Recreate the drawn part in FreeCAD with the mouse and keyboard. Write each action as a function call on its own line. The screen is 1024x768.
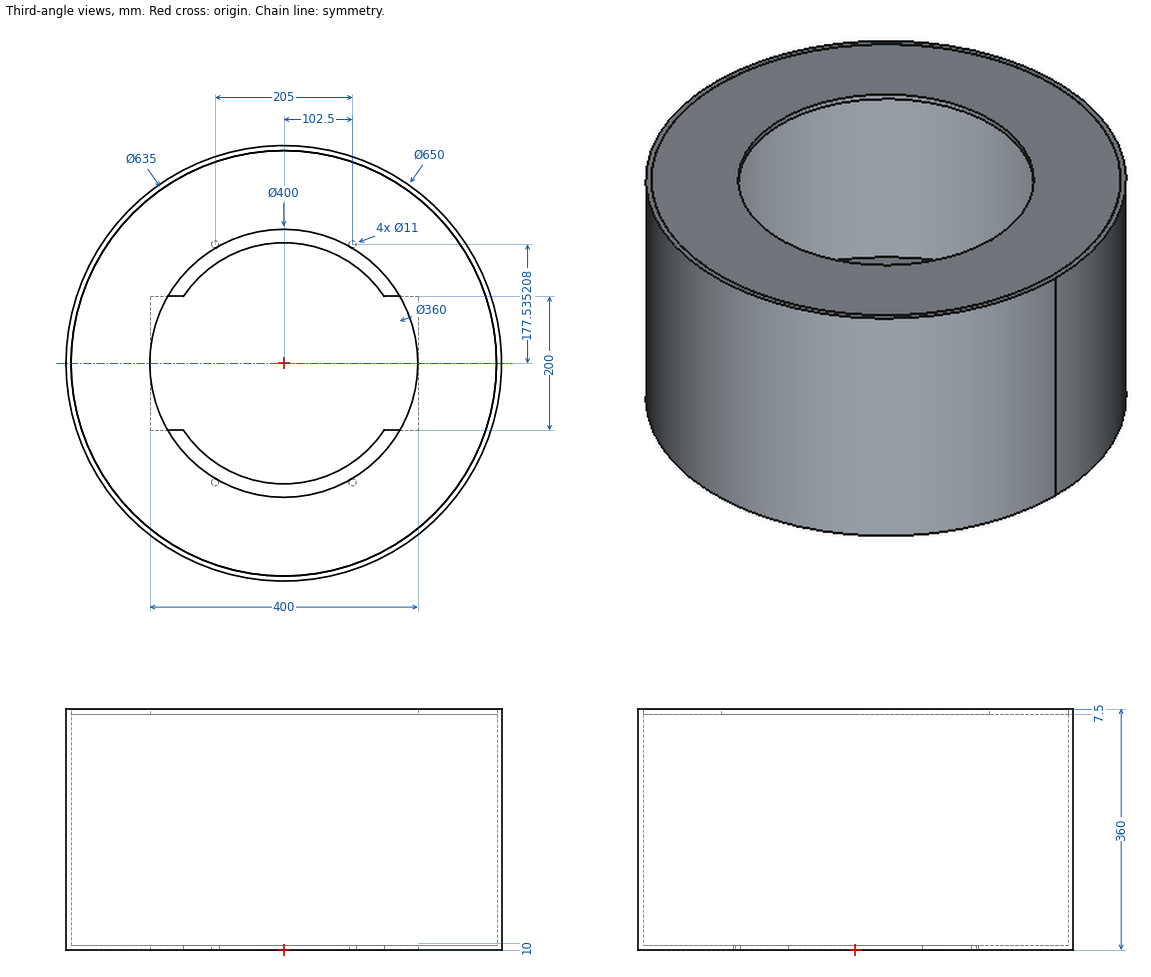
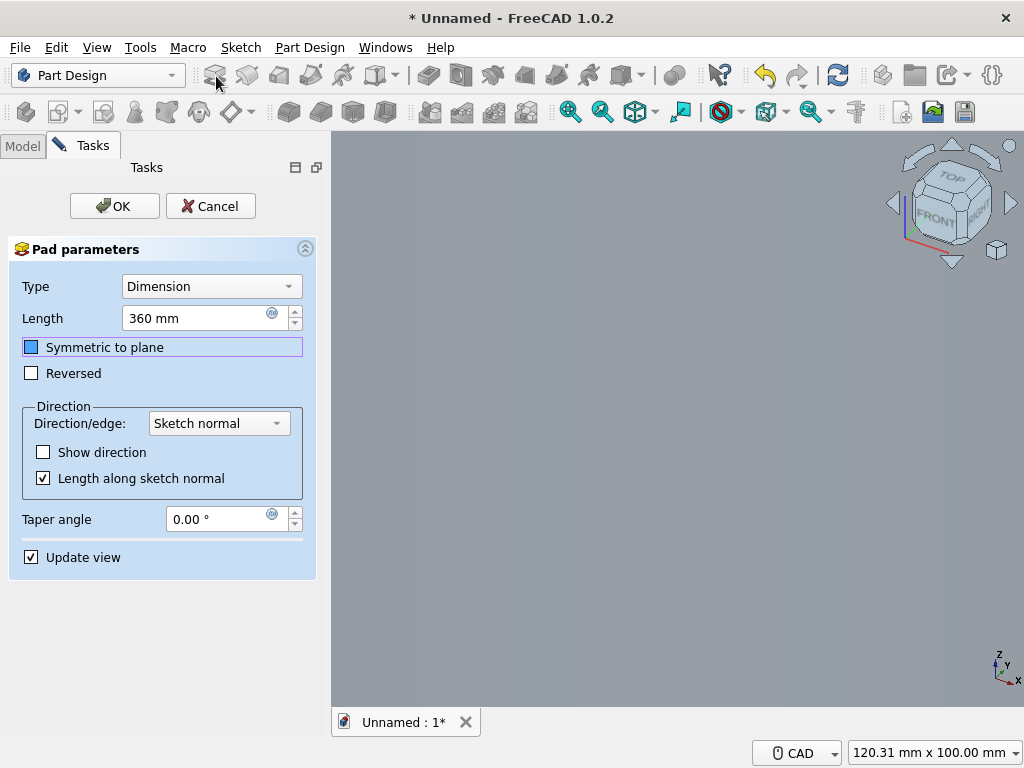
click(115, 206)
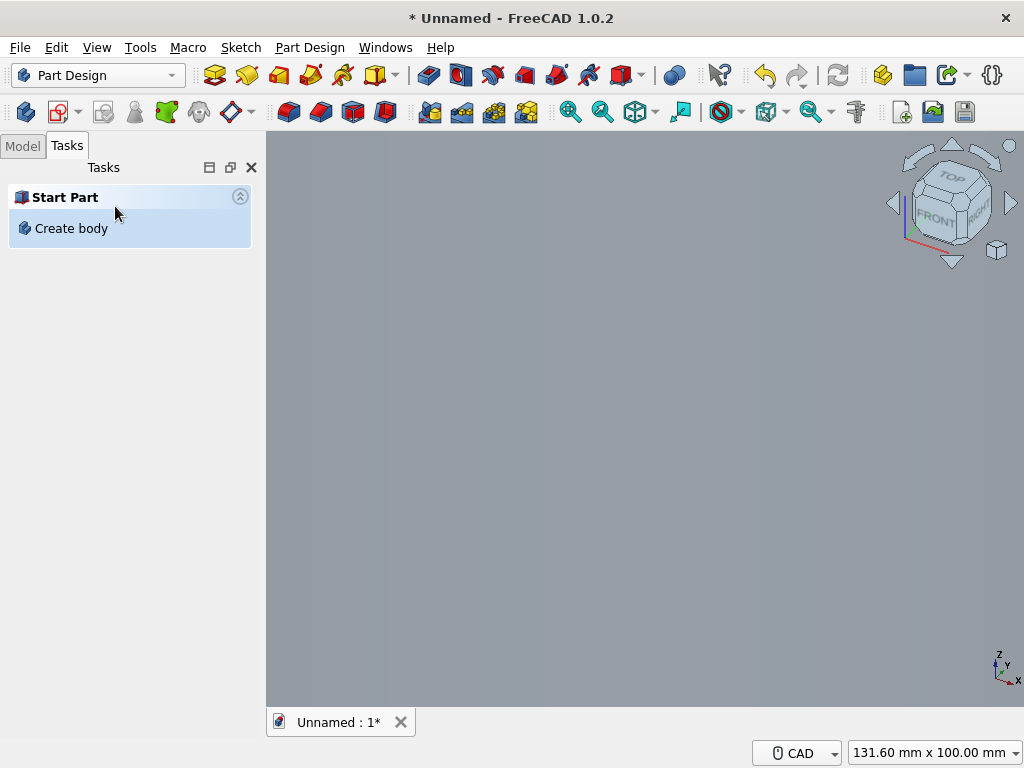
click(572, 112)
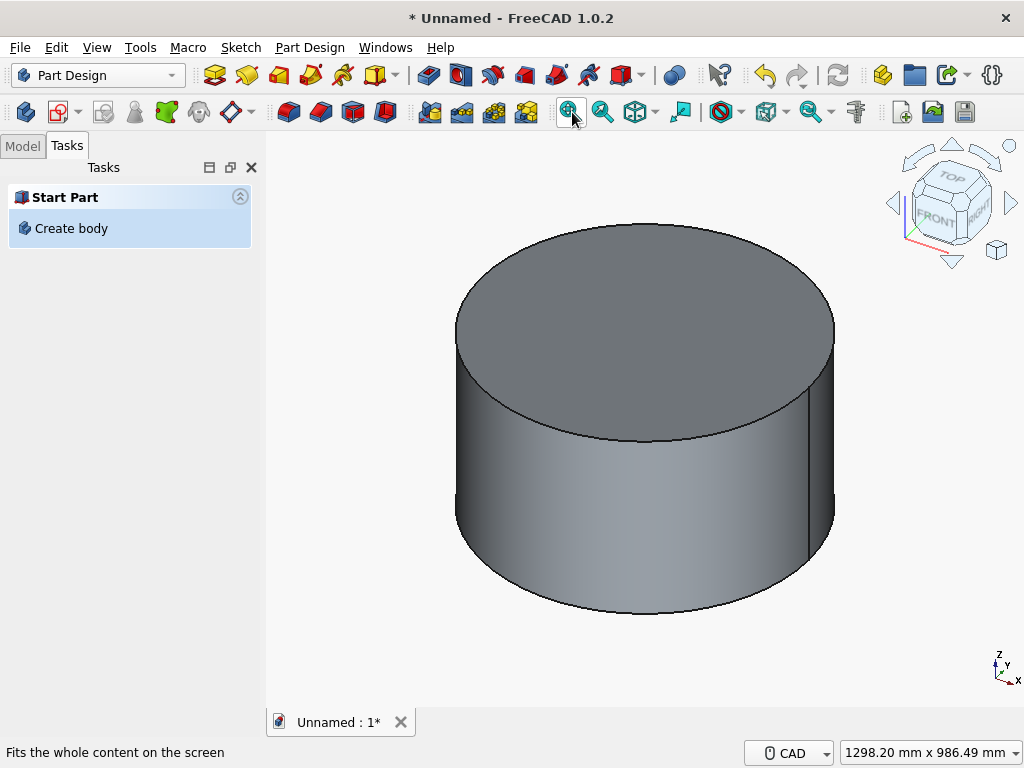
click(58, 112)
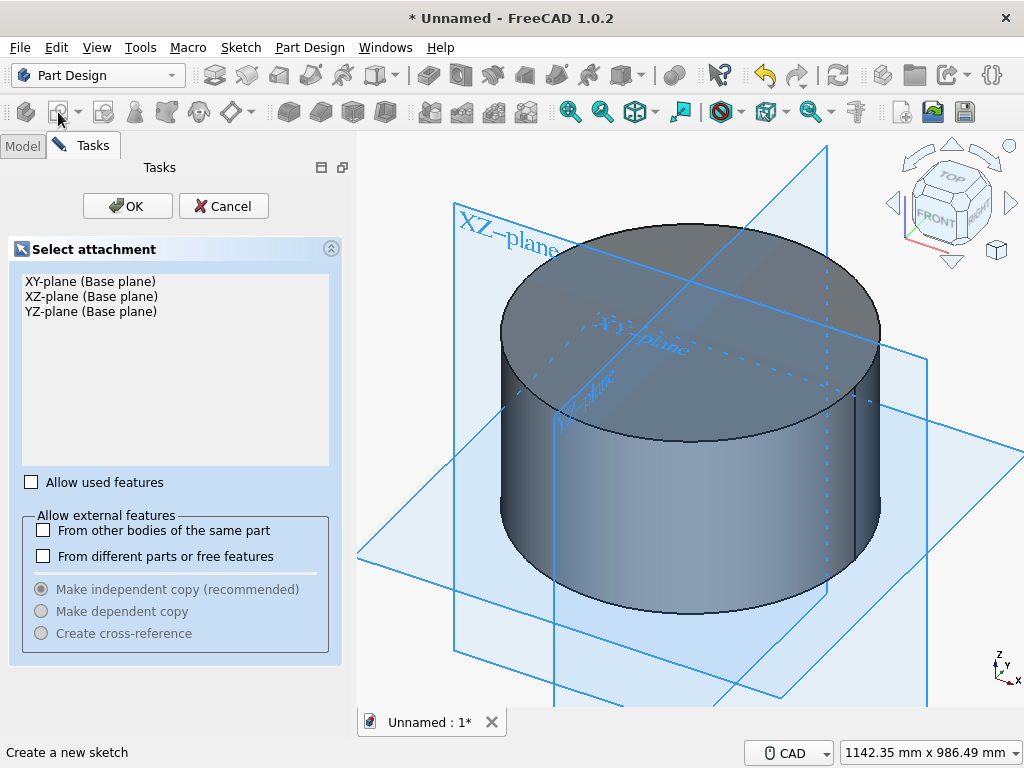
click(82, 282)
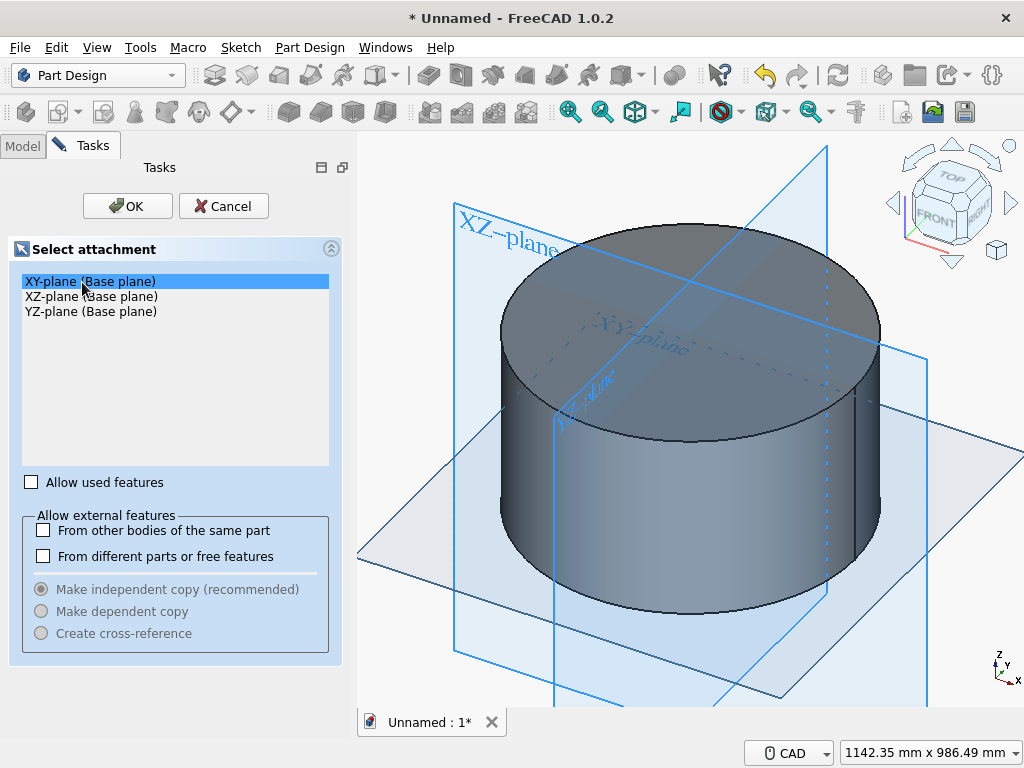
click(128, 206)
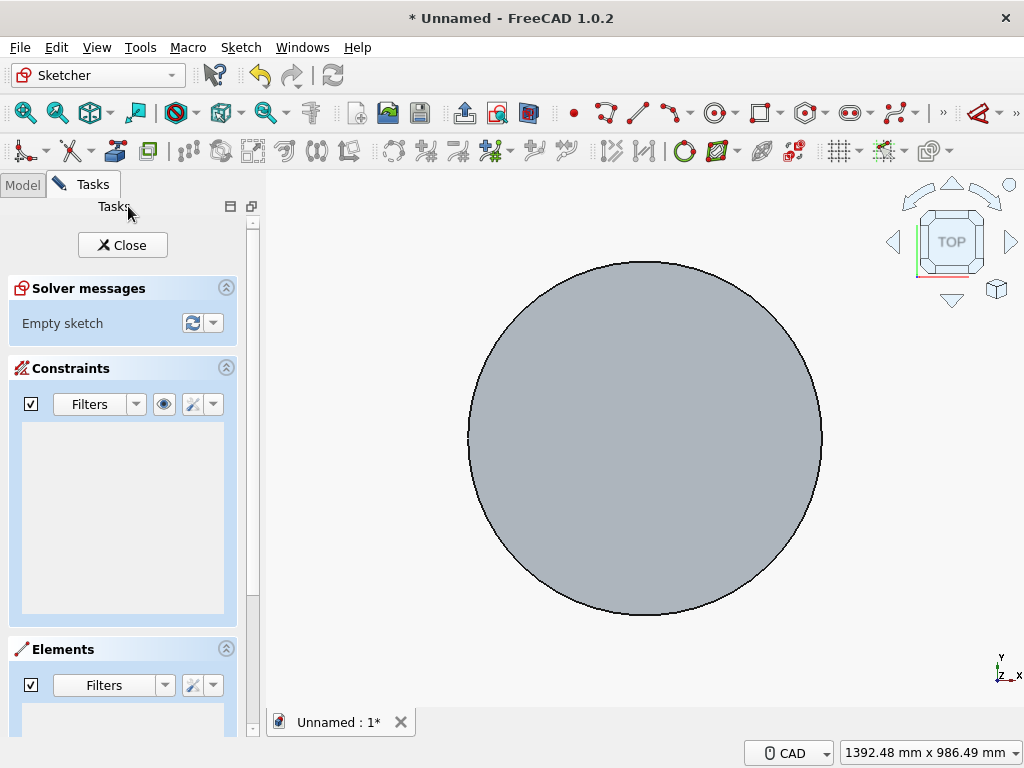
click(530, 114)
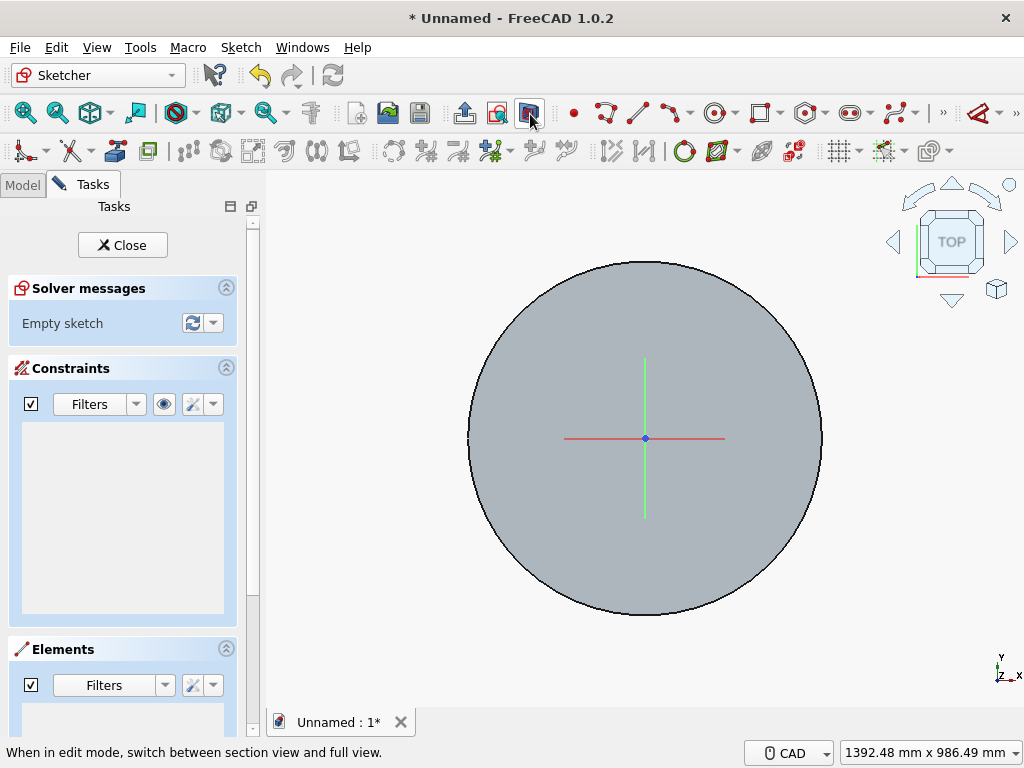
scroll(728, 438, up, 3)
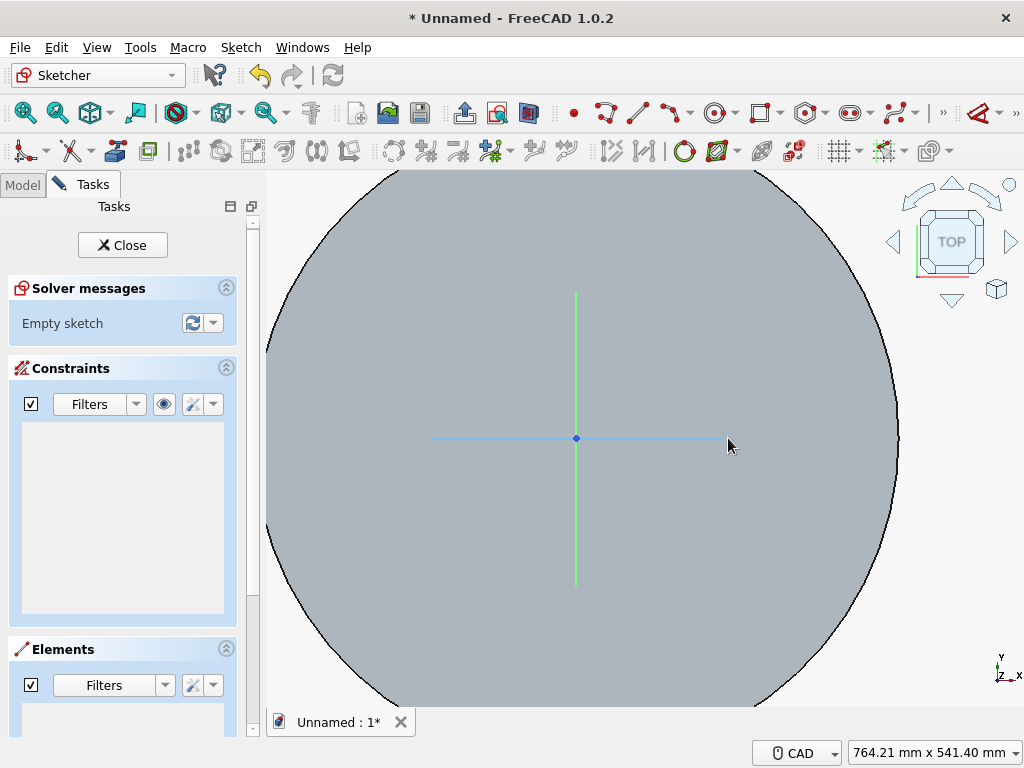
click(716, 114)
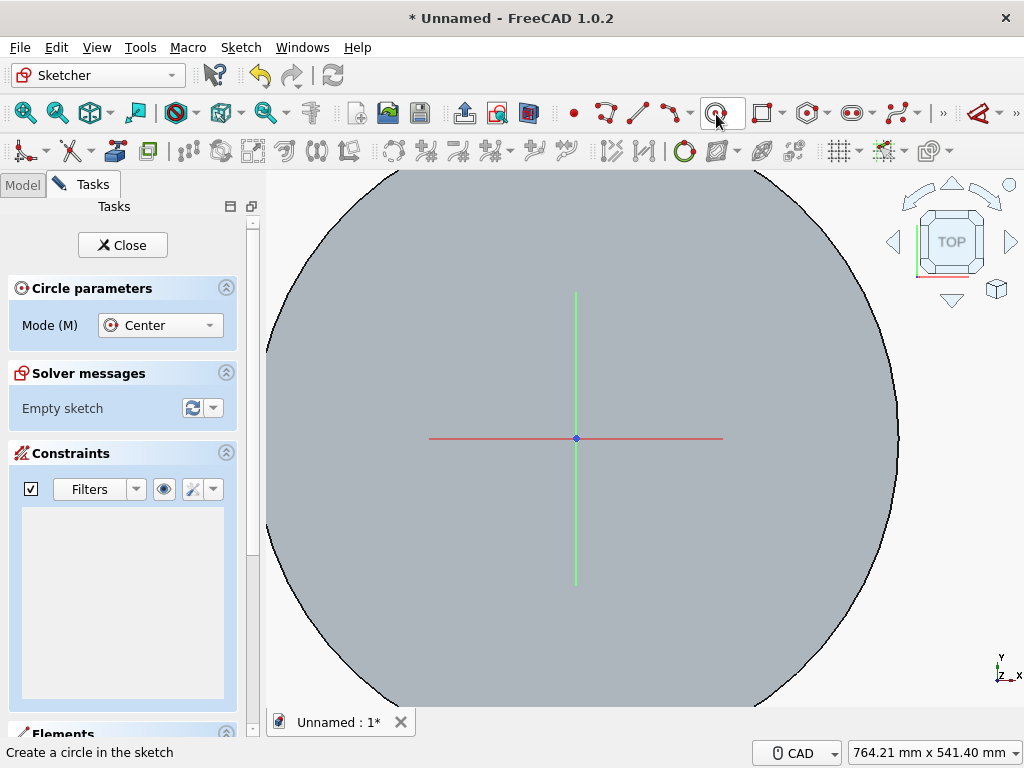
click(576, 438)
click(703, 312)
key(Escape)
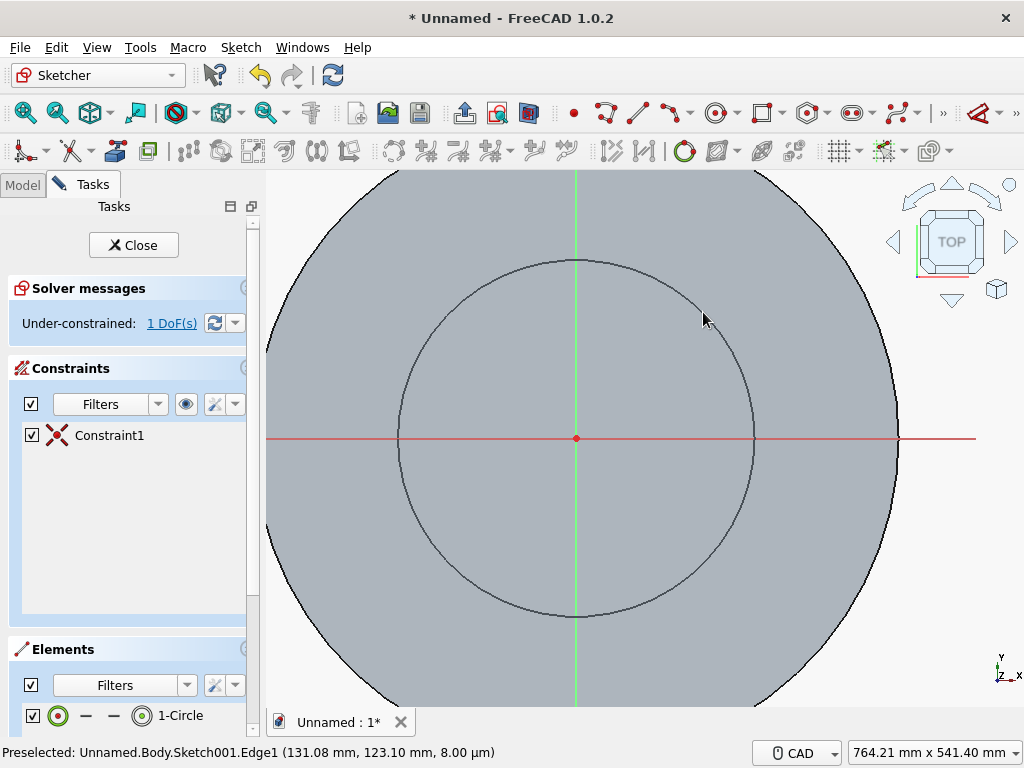
click(978, 114)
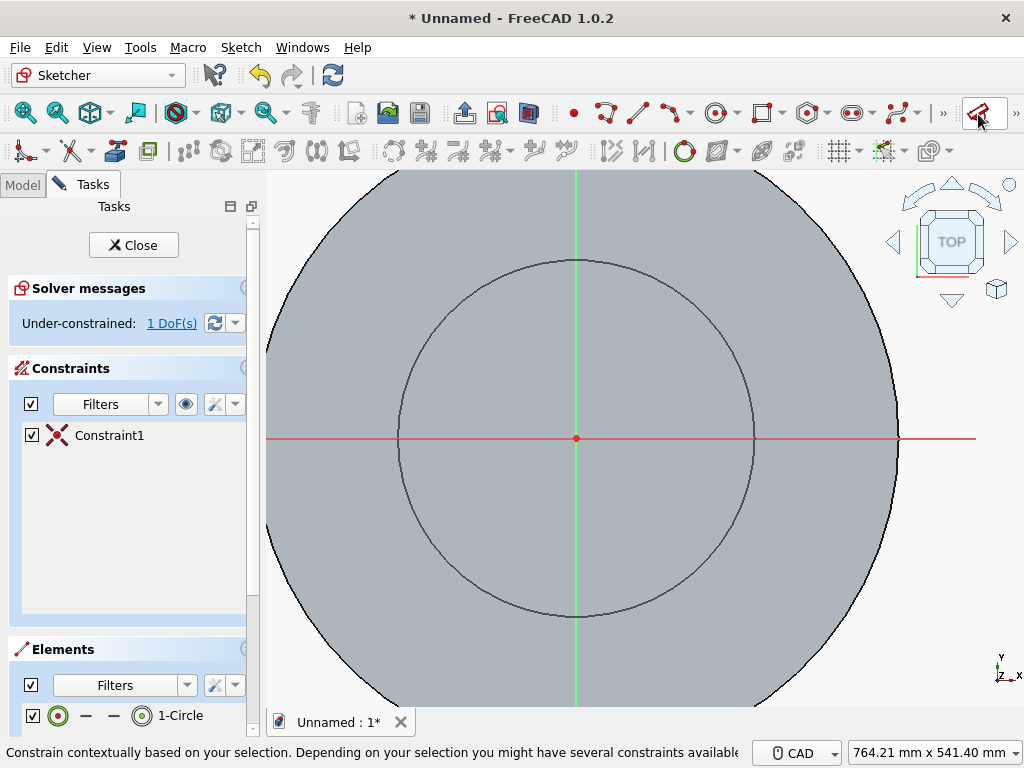
click(702, 312)
click(725, 289)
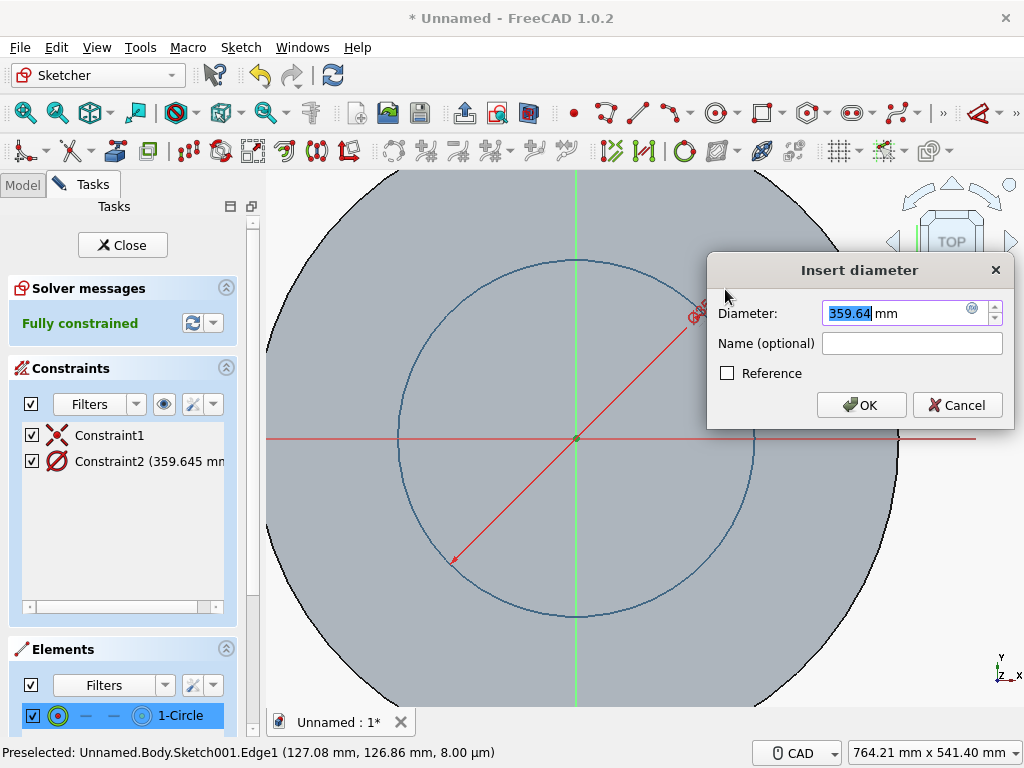
text(360)
key(Return)
key(Escape)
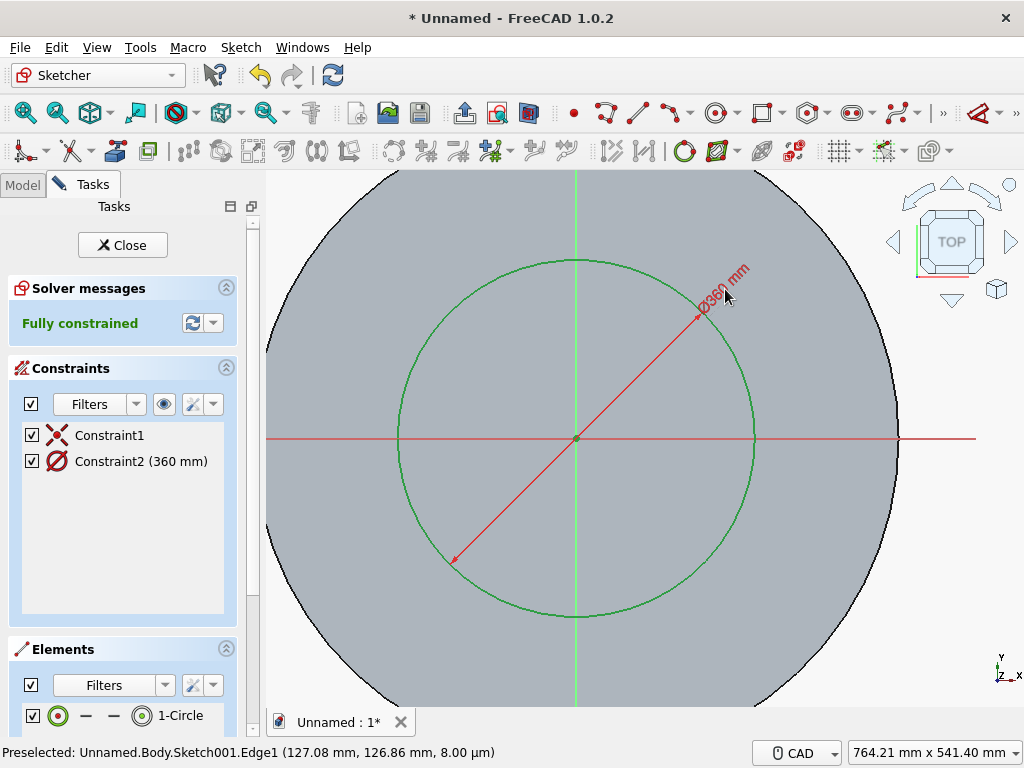
click(123, 245)